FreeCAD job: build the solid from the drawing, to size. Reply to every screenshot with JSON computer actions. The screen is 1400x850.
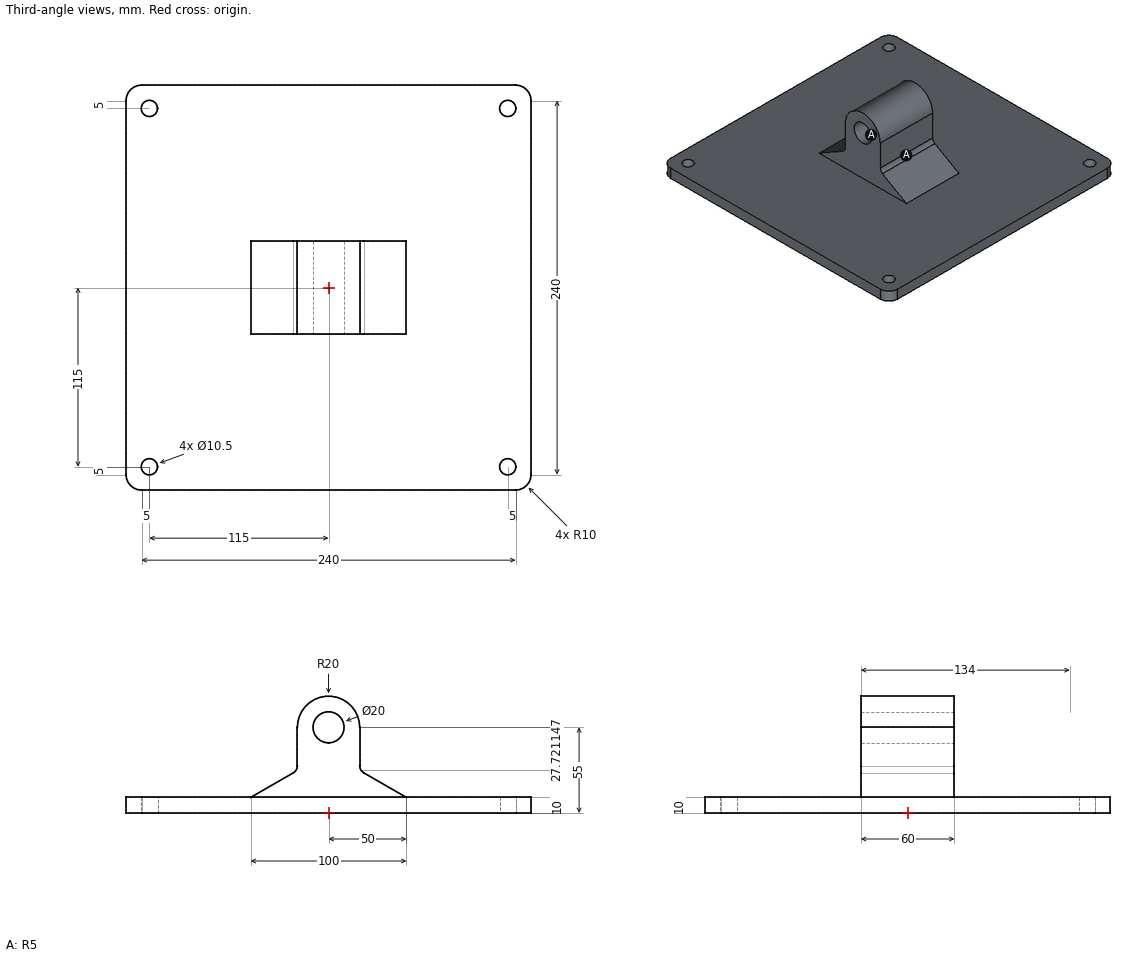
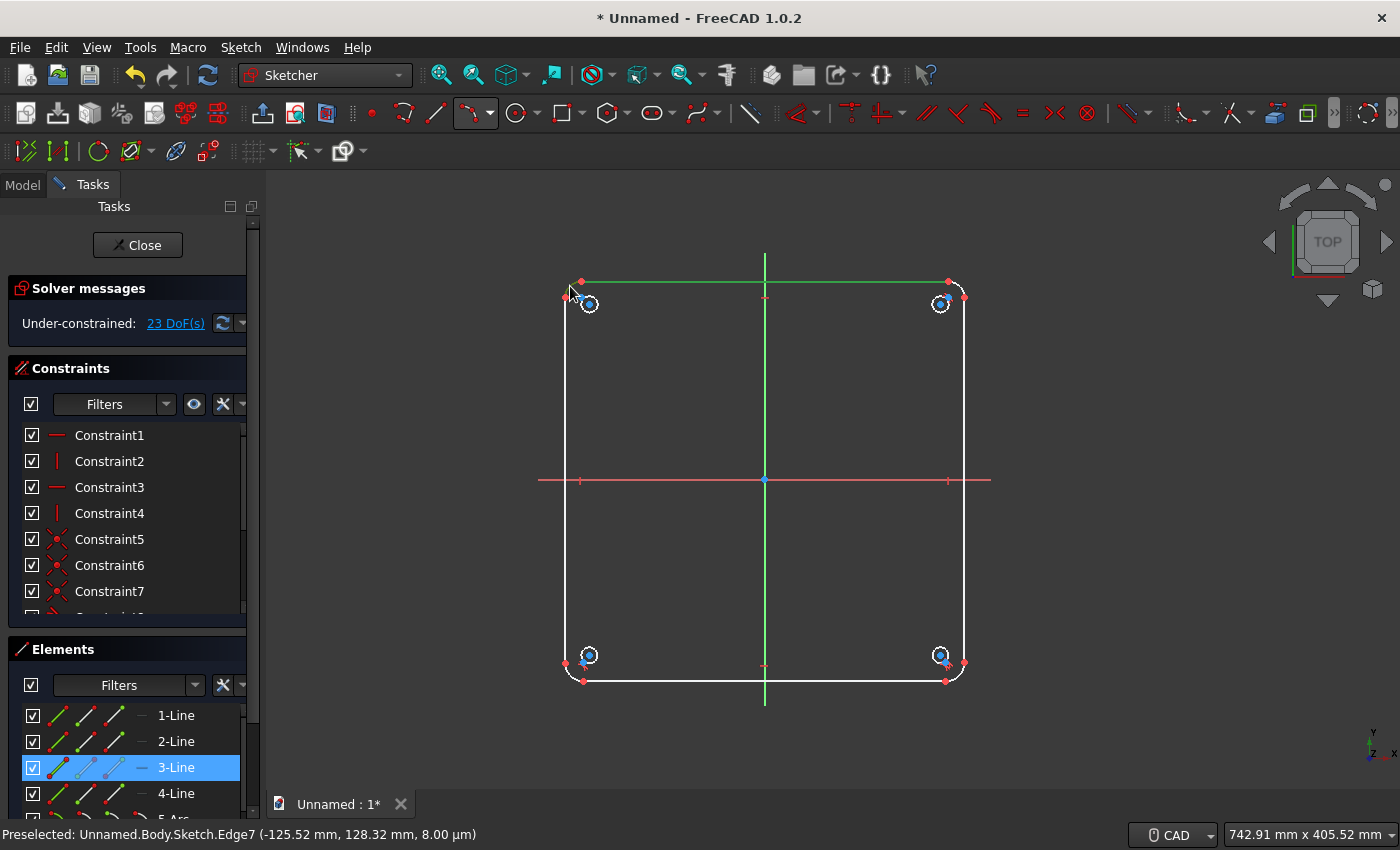
{"action": "left_click", "coordinate": [992, 114]}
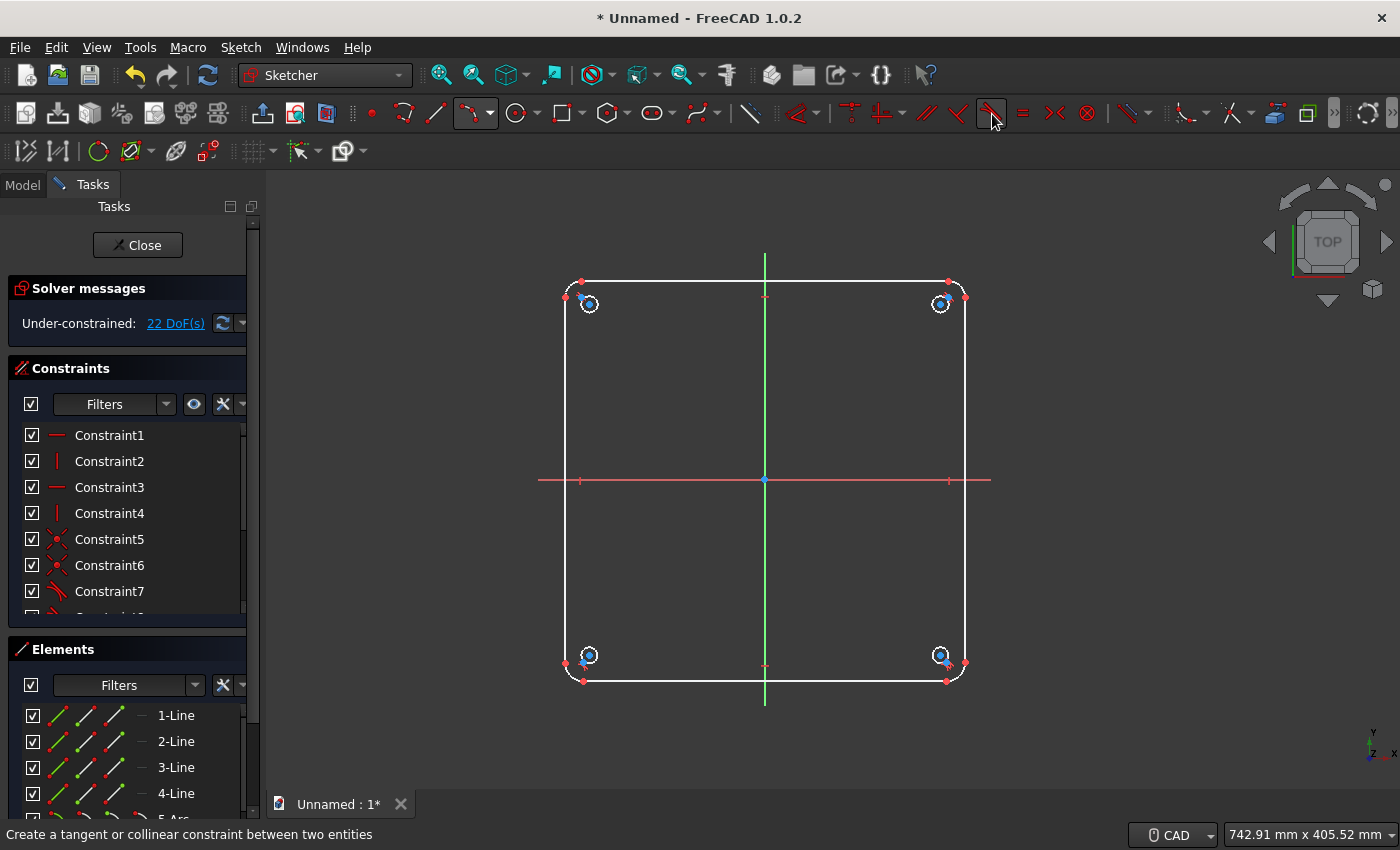
{"action": "left_click", "coordinate": [565, 407]}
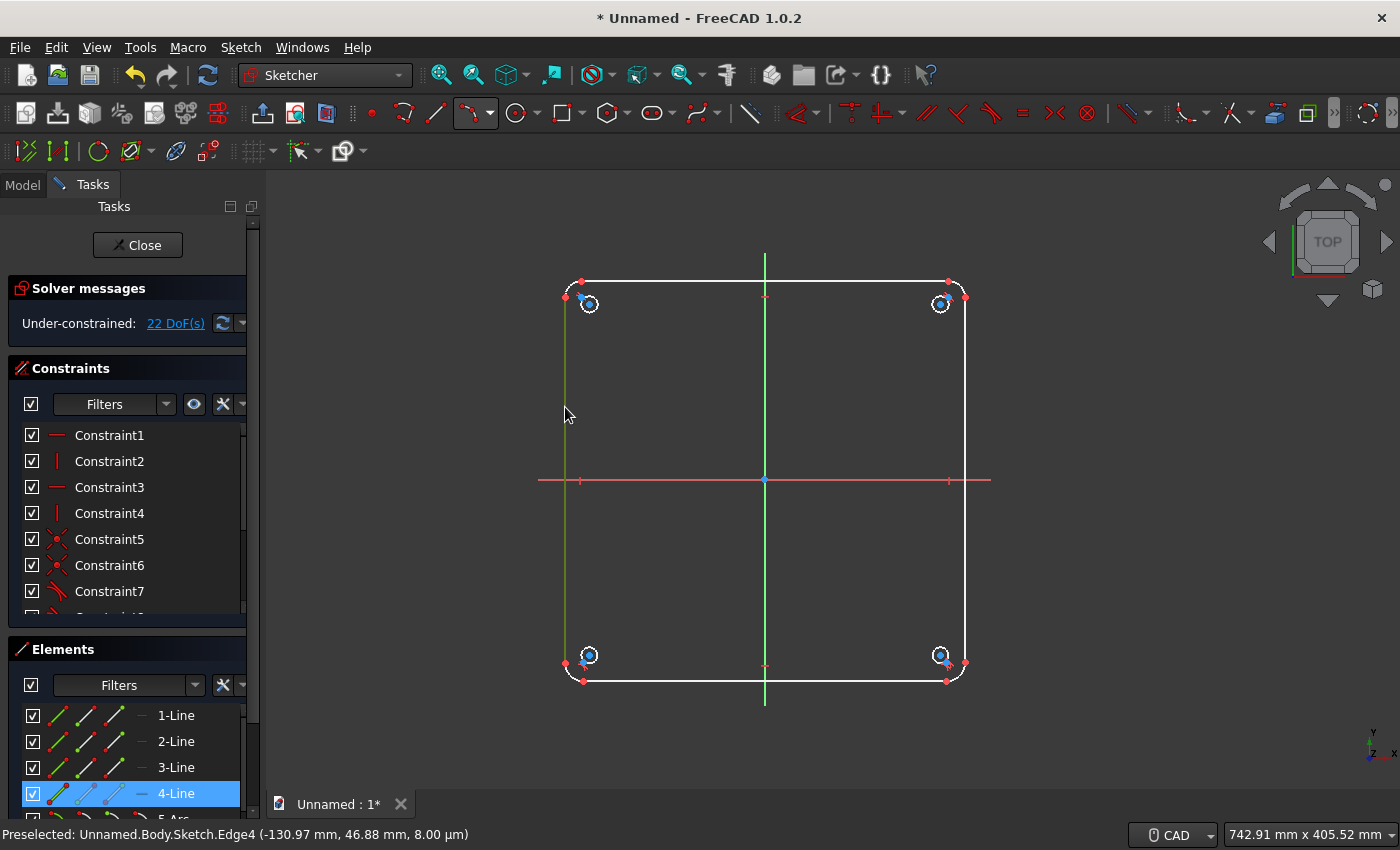
{"action": "left_click", "coordinate": [570, 286]}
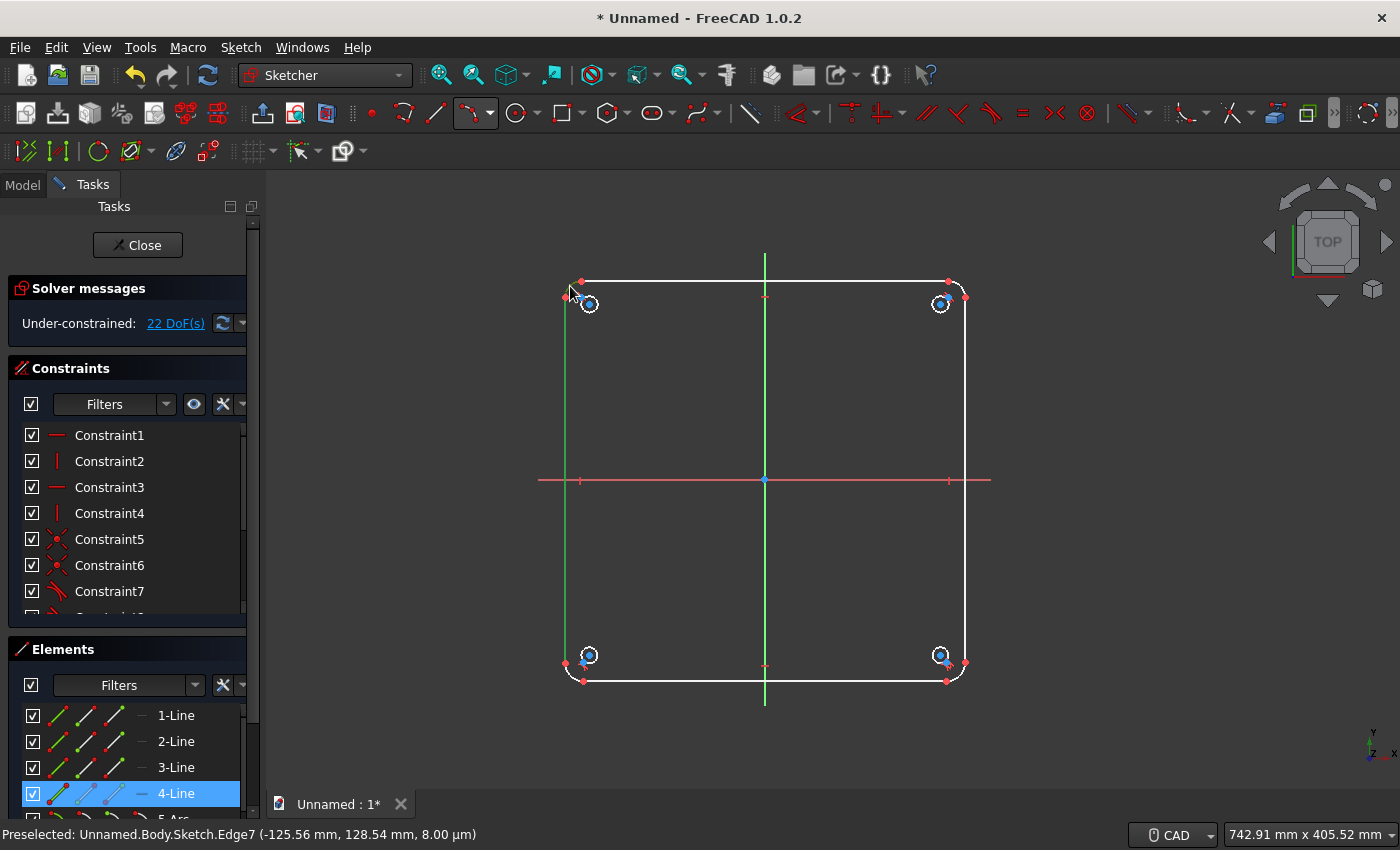
{"action": "left_click", "coordinate": [992, 114]}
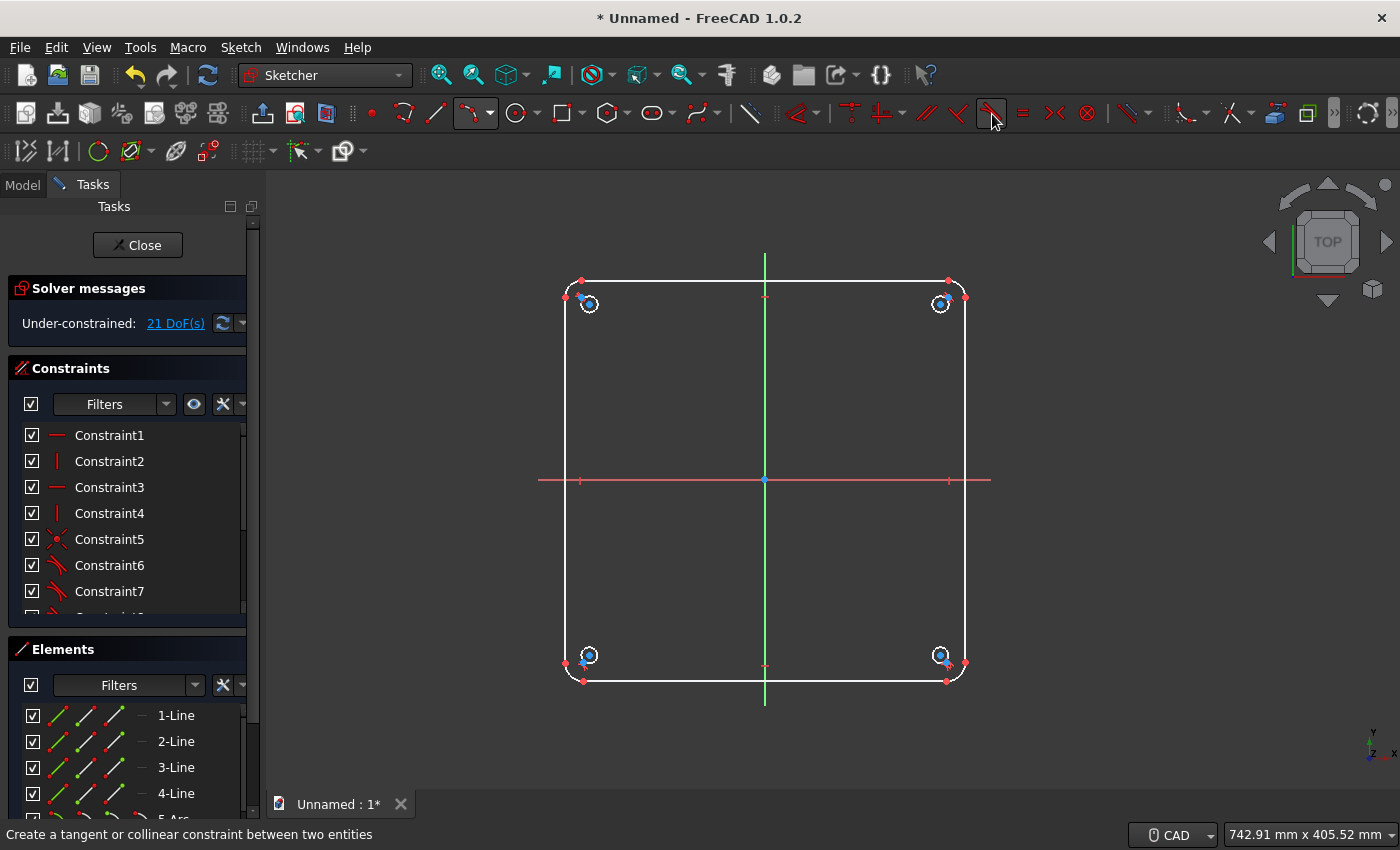
{"action": "left_click", "coordinate": [565, 407]}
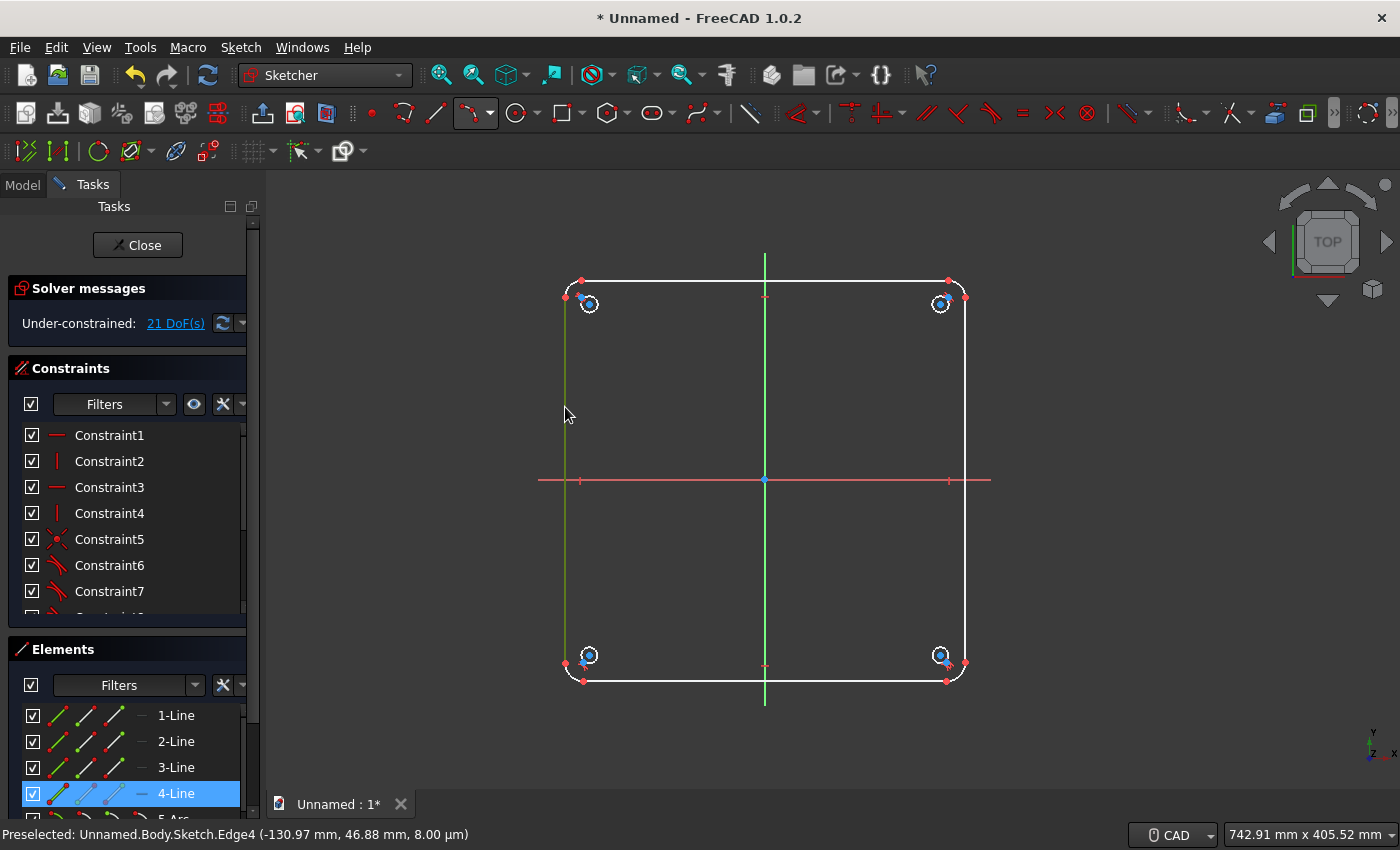
{"action": "left_click", "coordinate": [571, 676]}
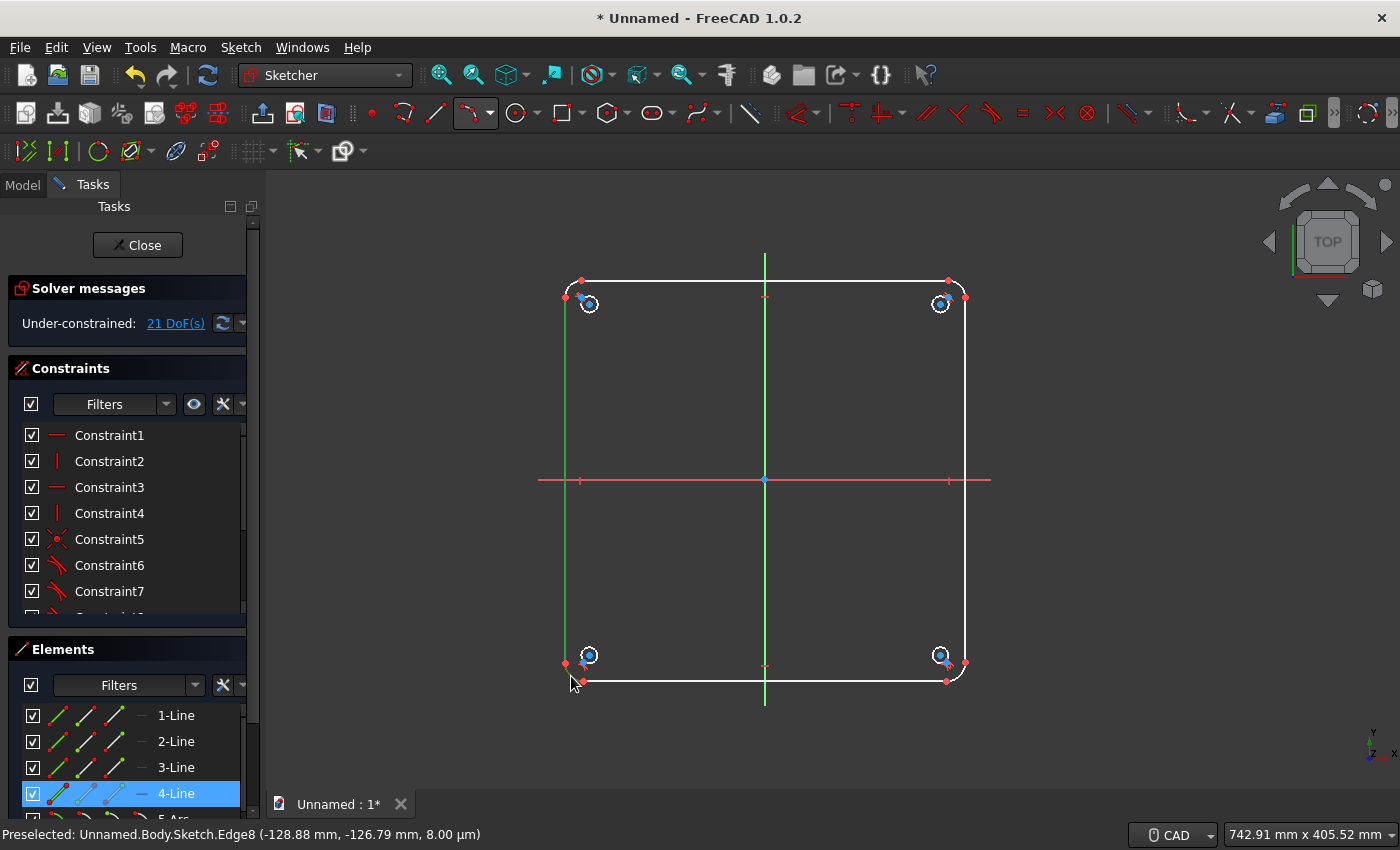
{"action": "left_click", "coordinate": [992, 114]}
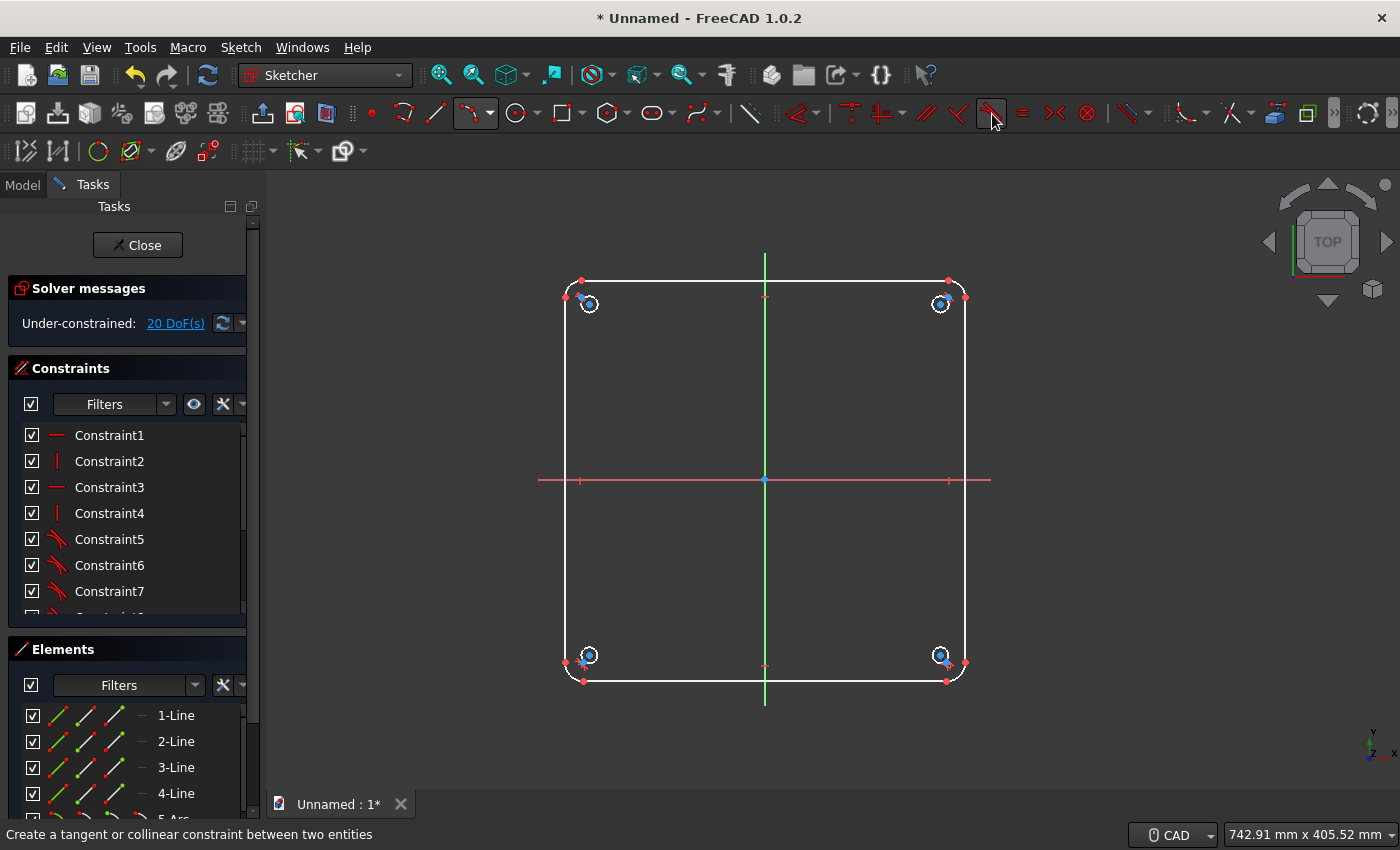
{"action": "left_click", "coordinate": [960, 676]}